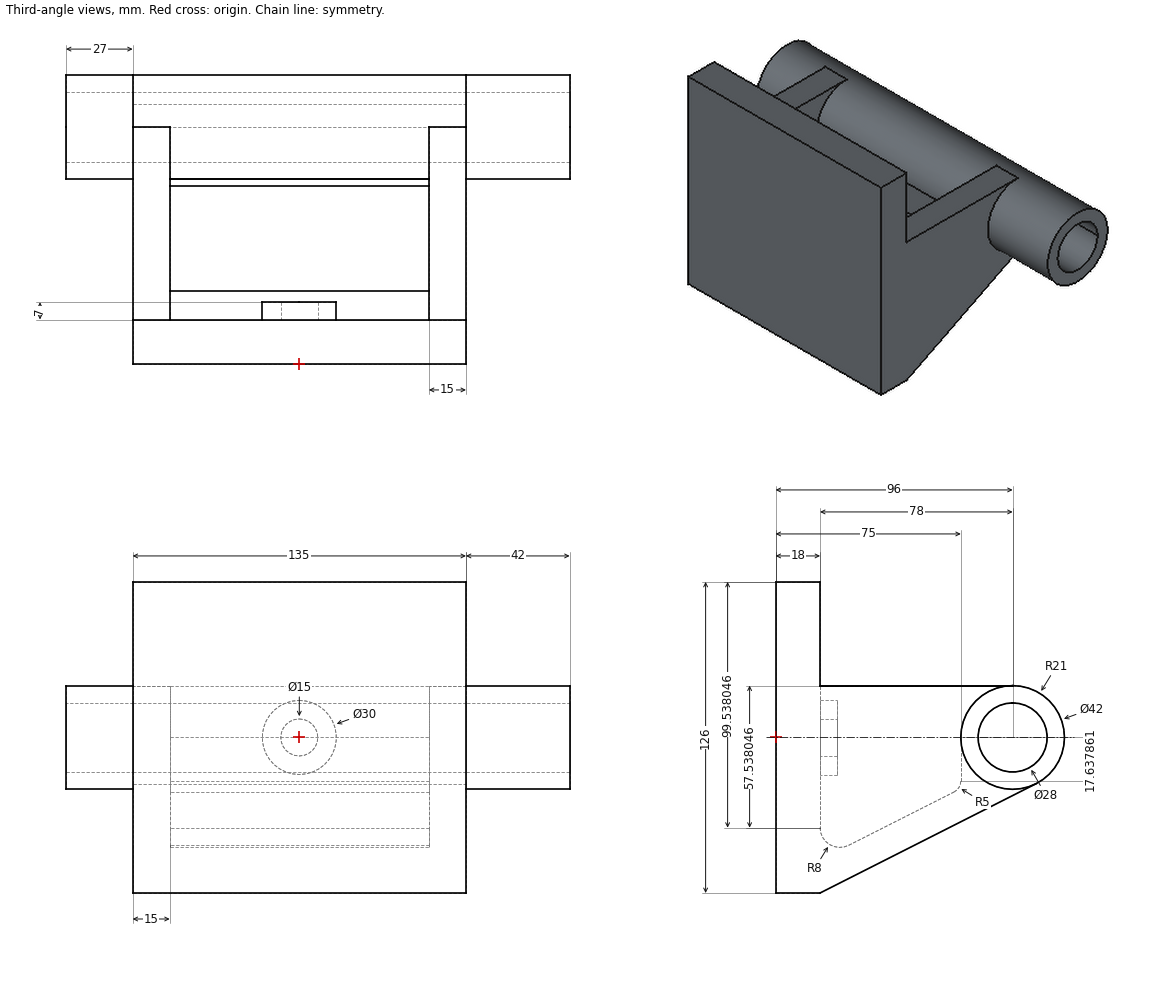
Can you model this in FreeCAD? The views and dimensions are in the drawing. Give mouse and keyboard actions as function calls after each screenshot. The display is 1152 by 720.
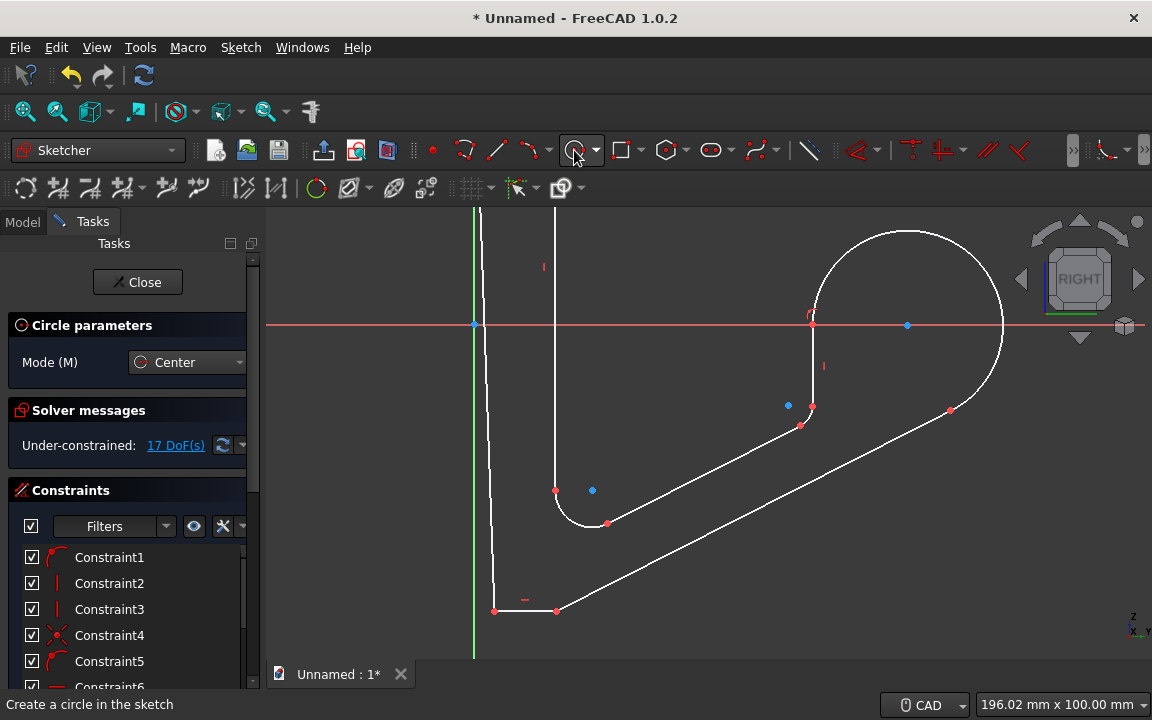
click(908, 325)
click(953, 280)
key(Escape)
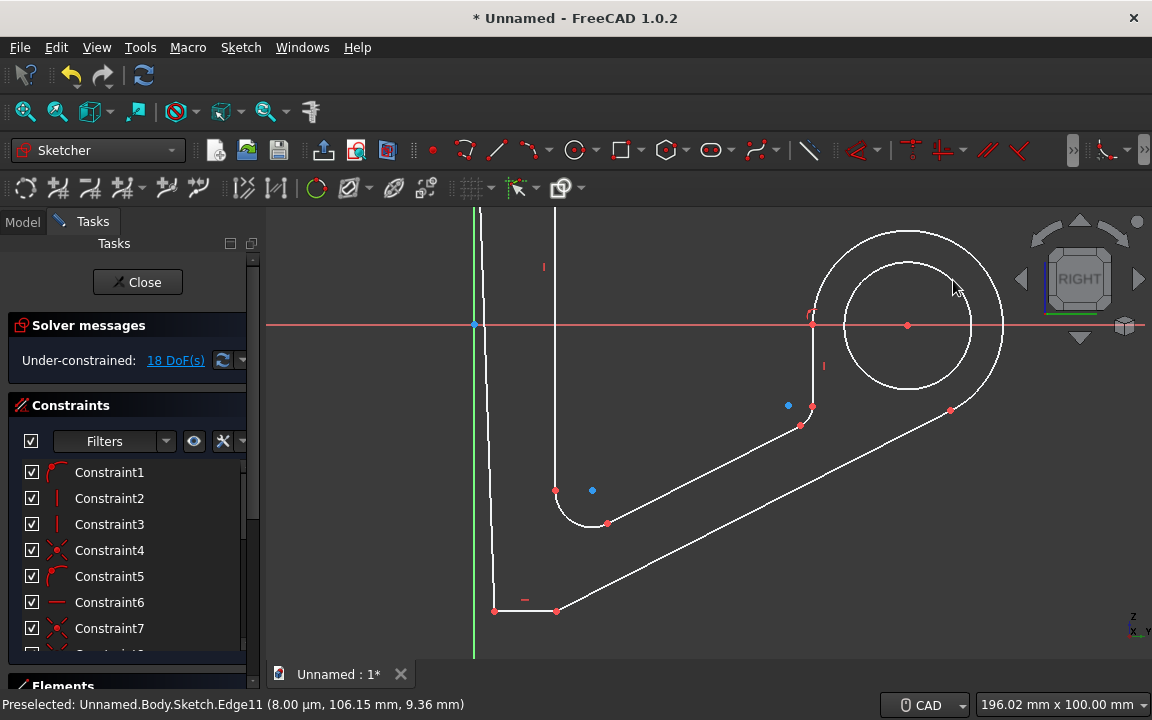
click(813, 349)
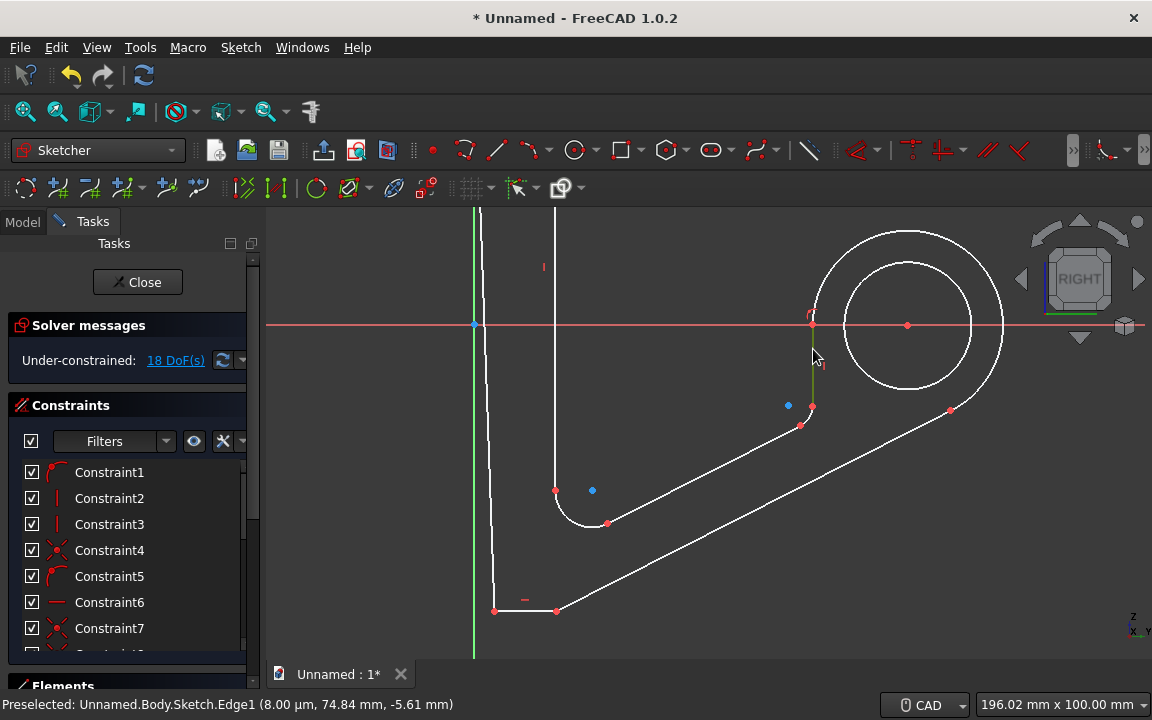
click(809, 418)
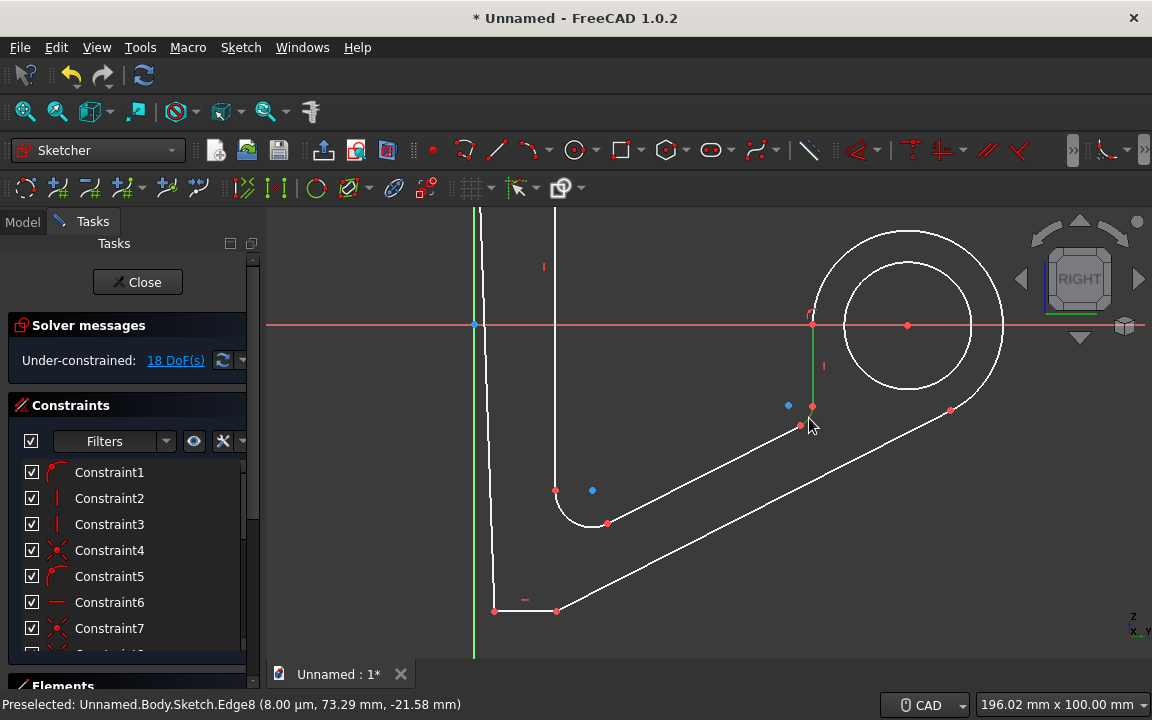
key(t)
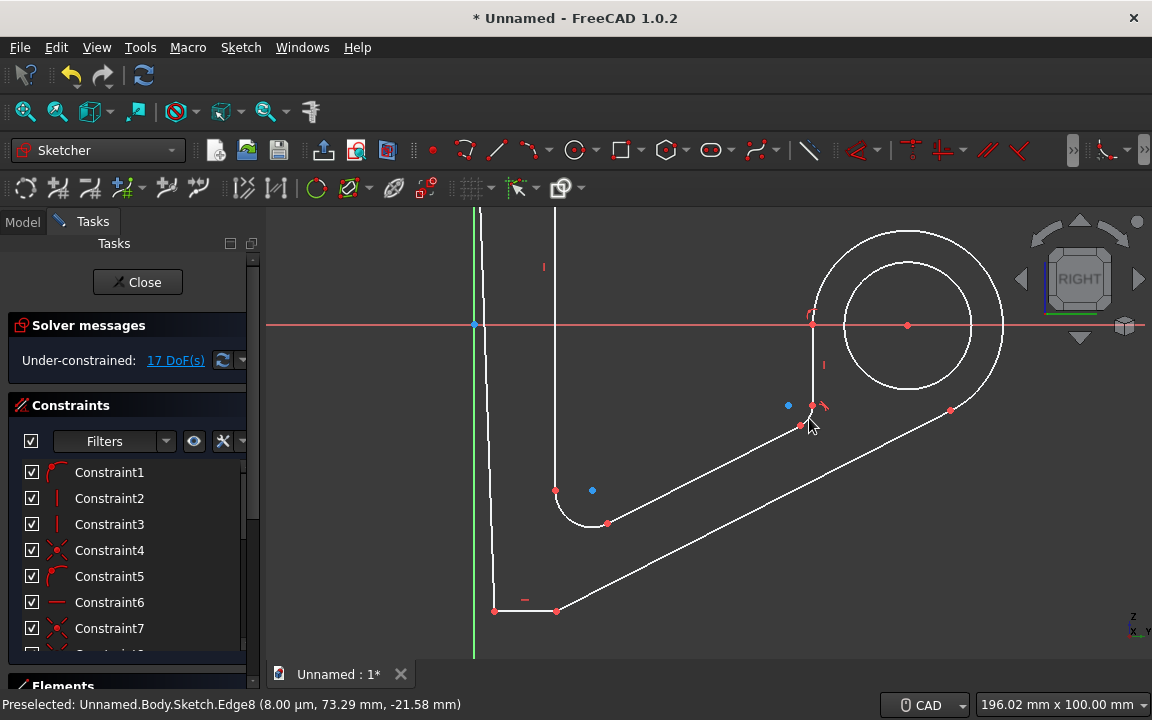
click(813, 349)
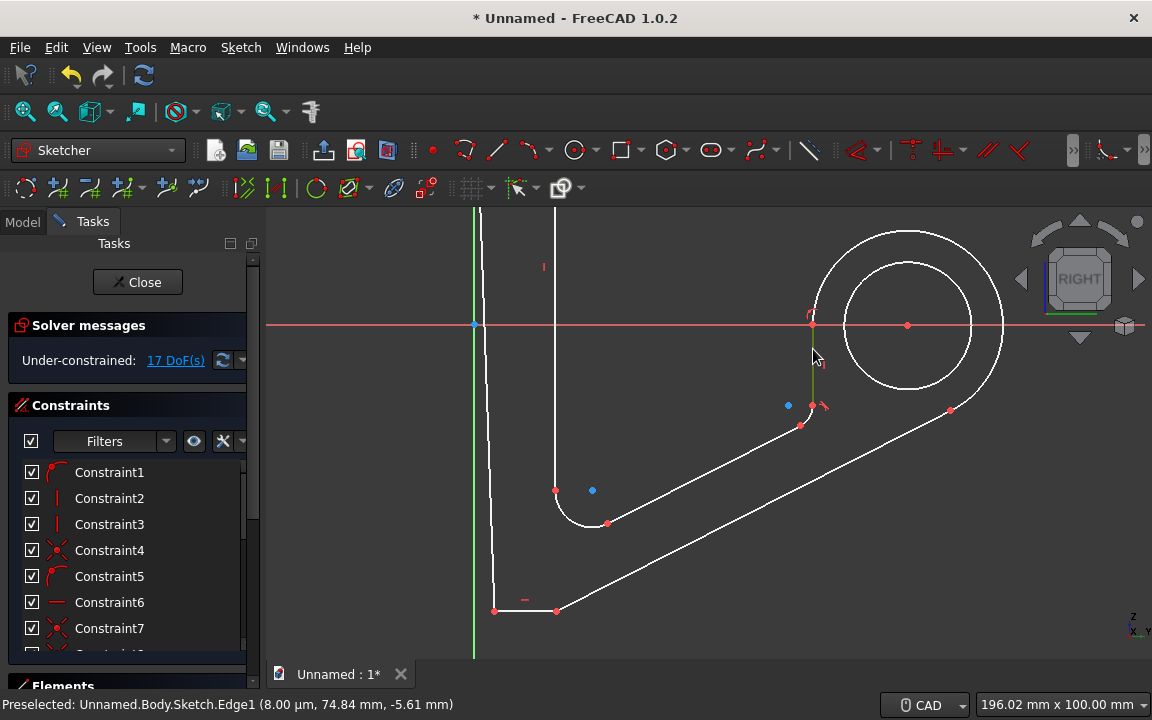
click(958, 245)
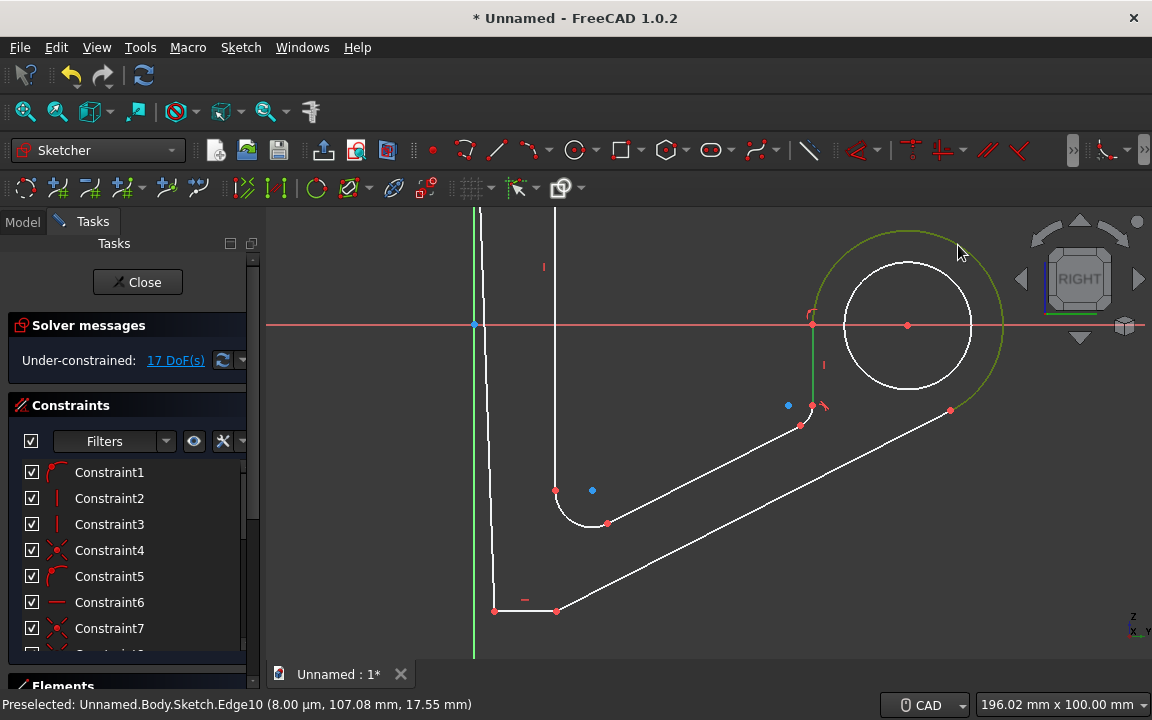
key(t)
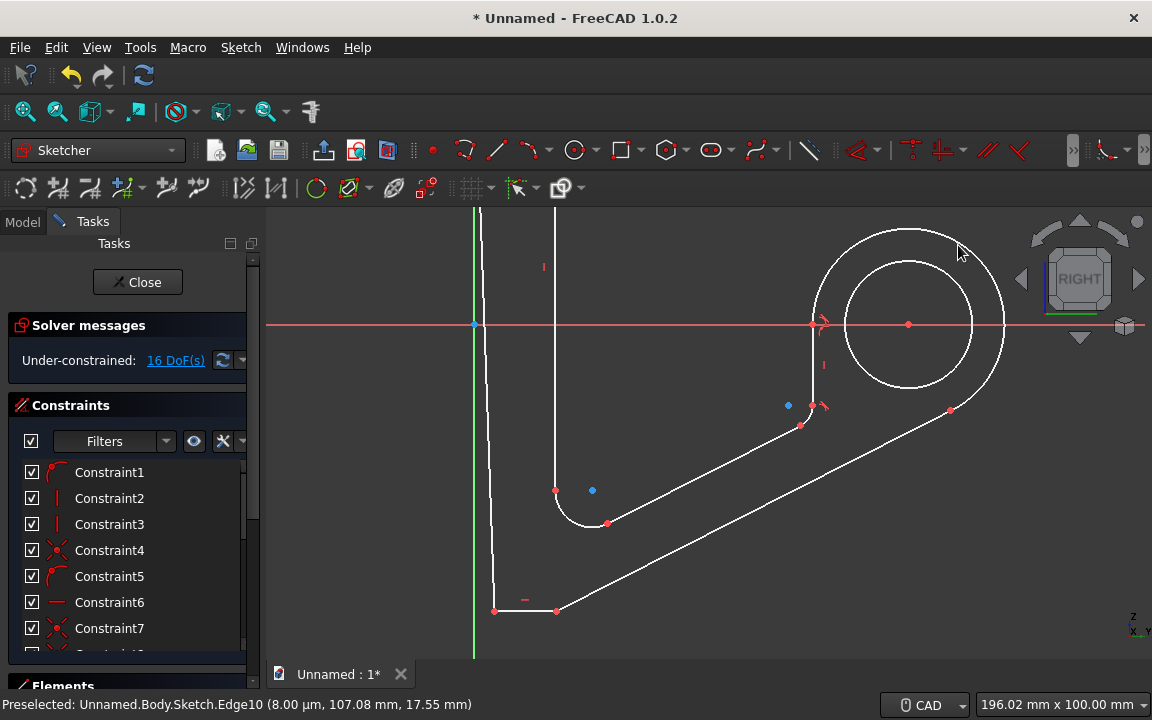
click(743, 455)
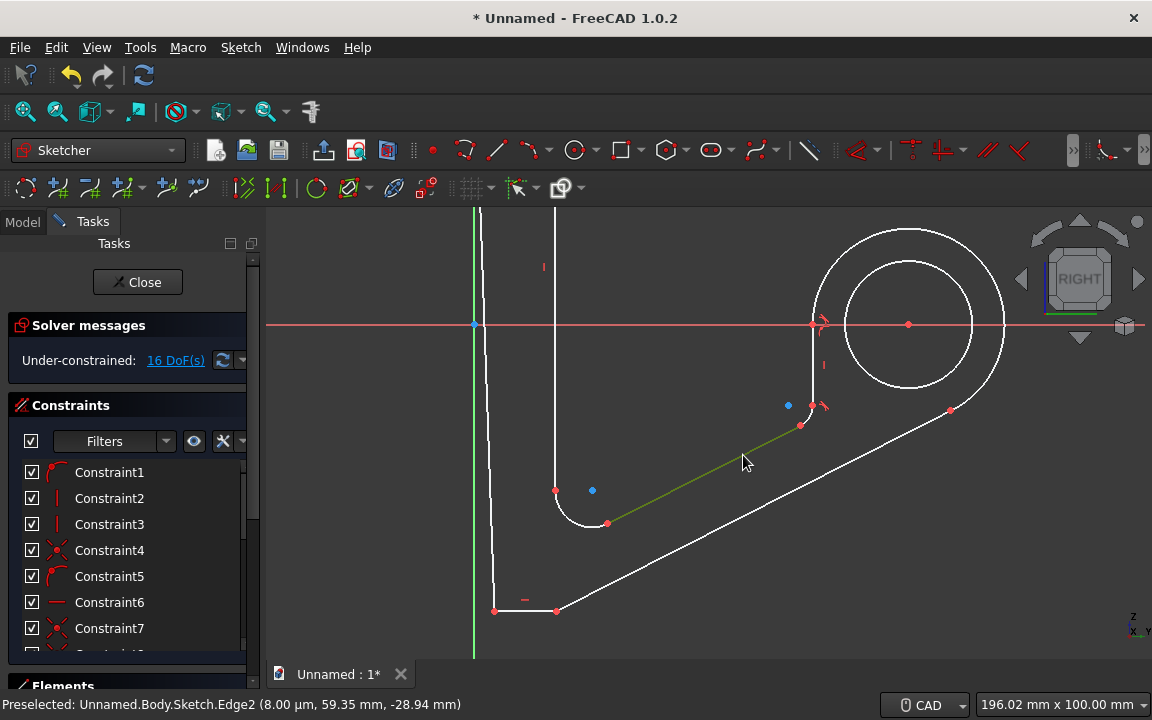
click(810, 417)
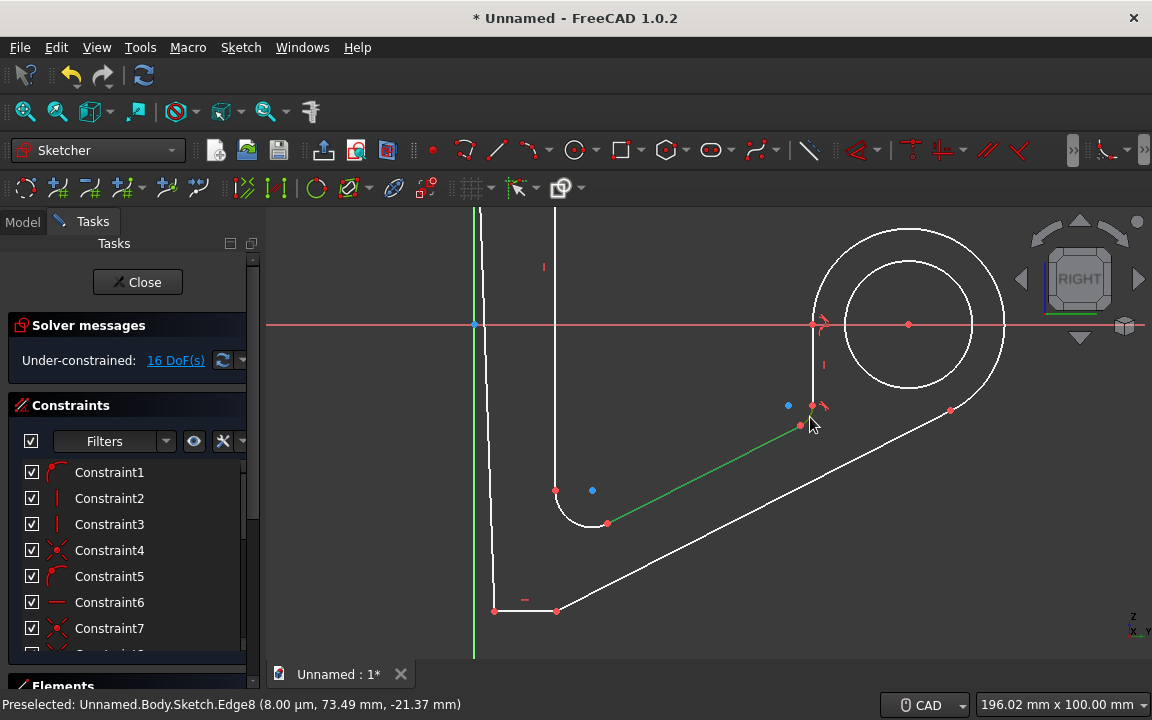
key(t)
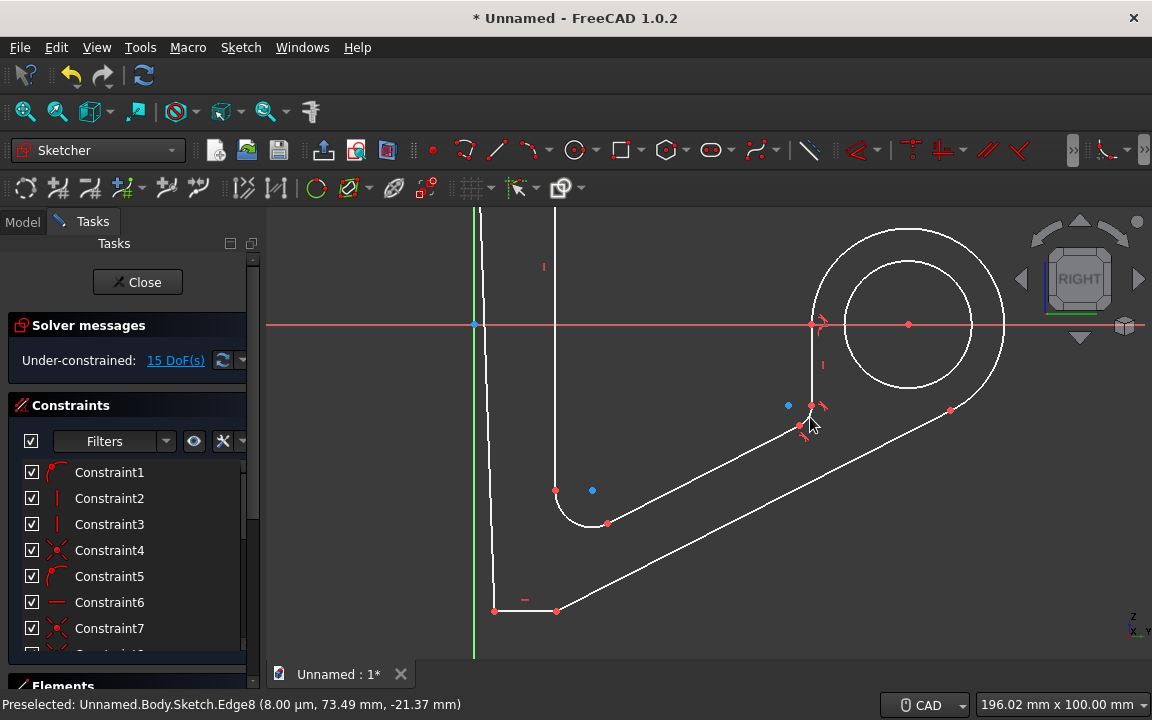
click(742, 455)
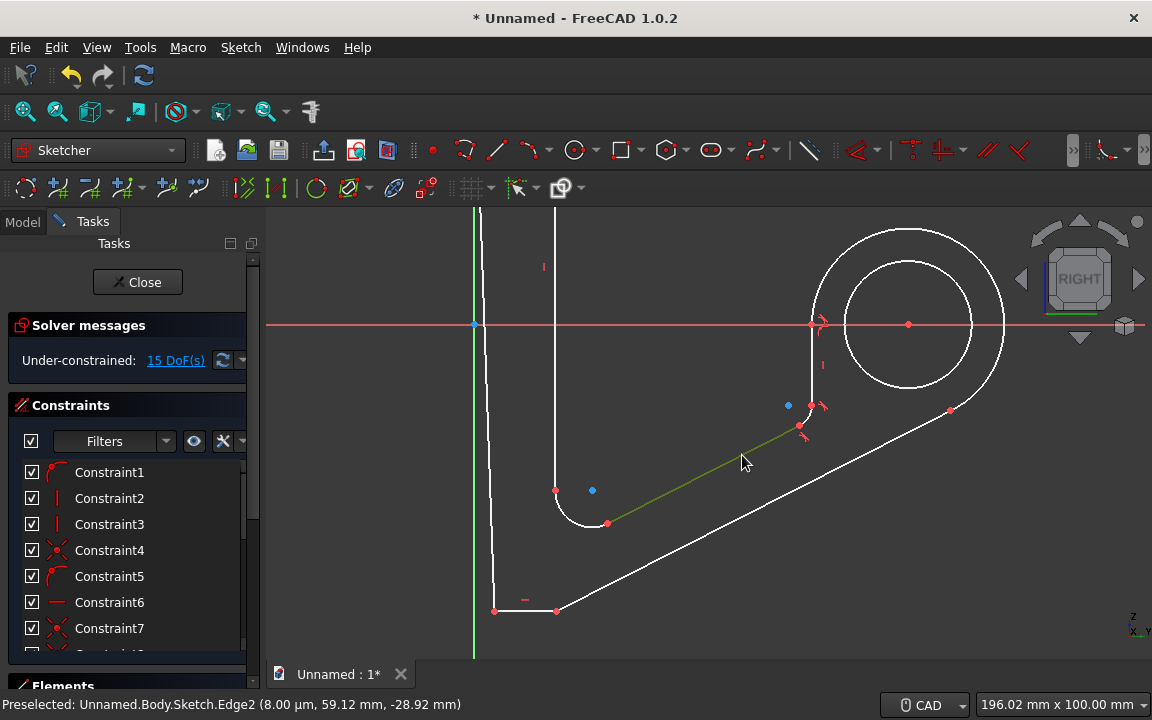
click(562, 512)